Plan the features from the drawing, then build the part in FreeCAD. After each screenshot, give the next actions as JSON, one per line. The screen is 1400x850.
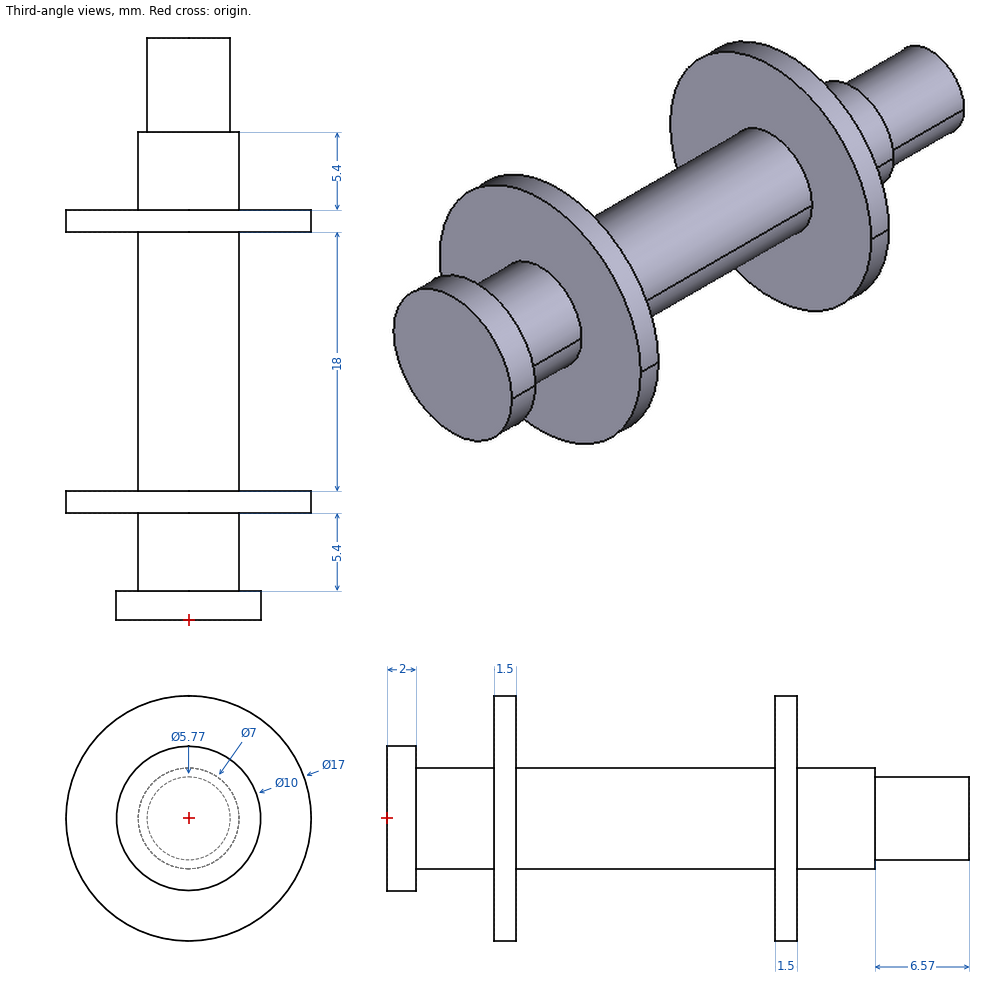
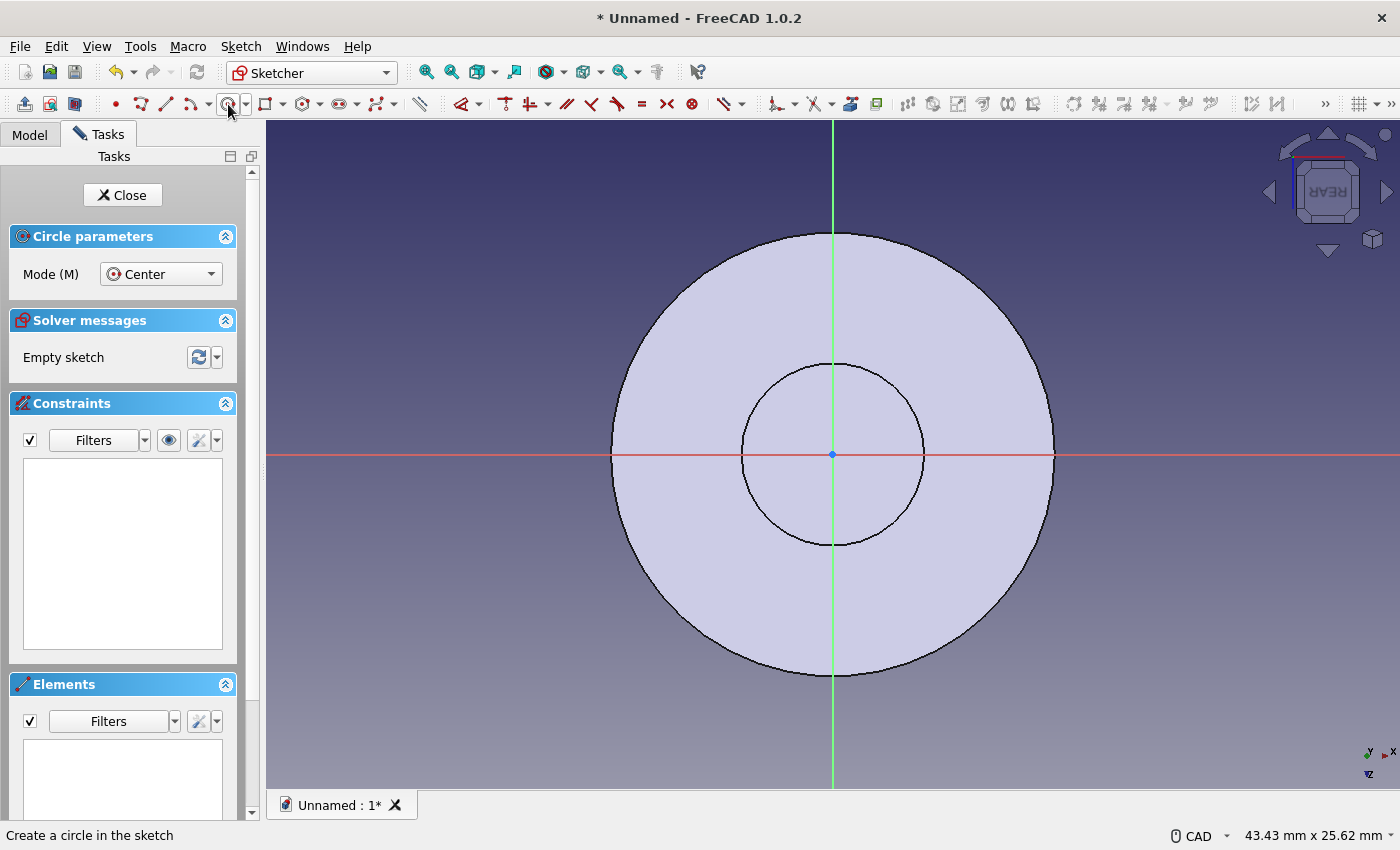
{"action": "left_click", "coordinate": [833, 455]}
{"action": "left_click", "coordinate": [990, 298]}
{"action": "key", "text": "Escape"}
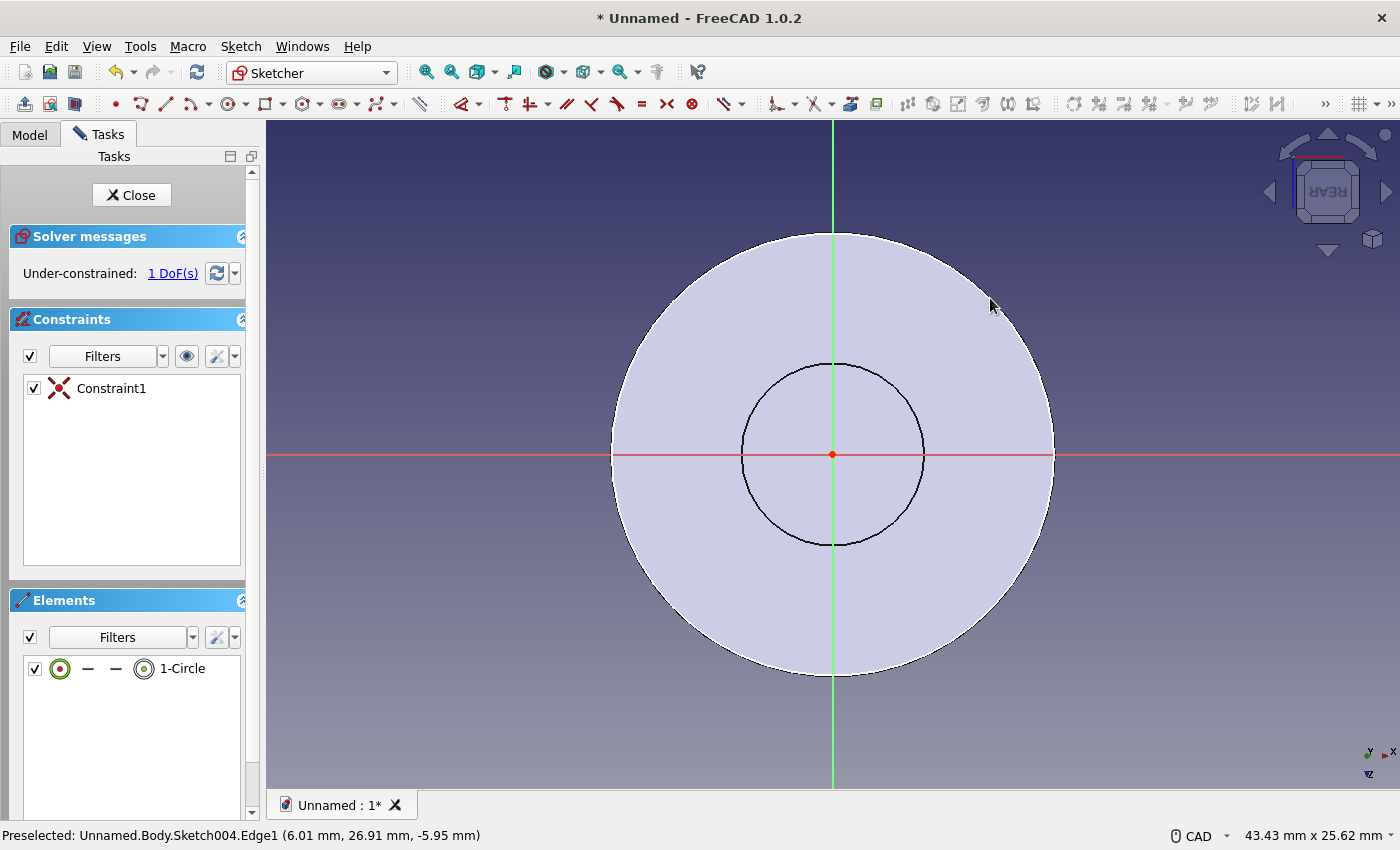
{"action": "left_click", "coordinate": [460, 104]}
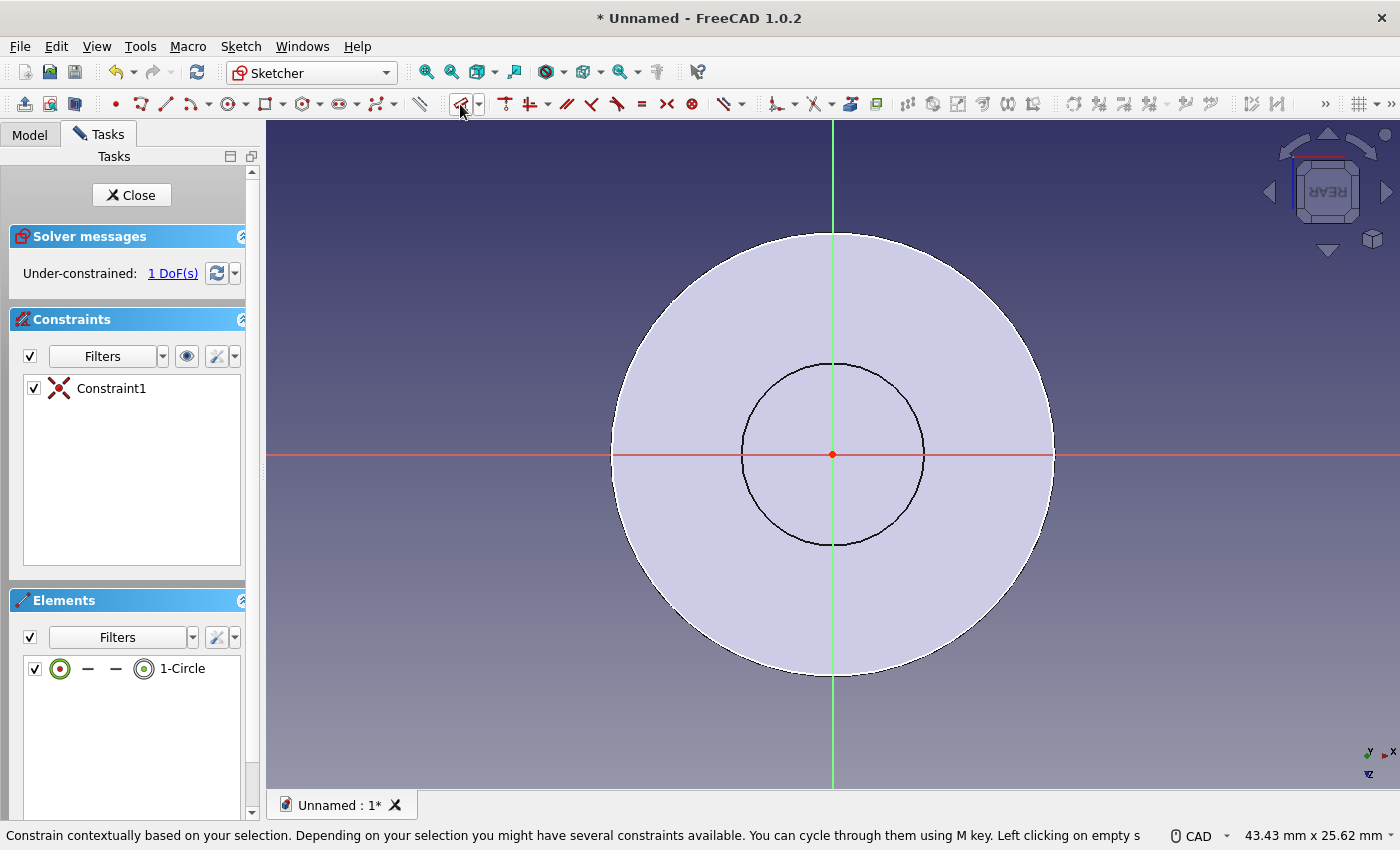
{"action": "left_click", "coordinate": [989, 298]}
{"action": "left_click", "coordinate": [1012, 275]}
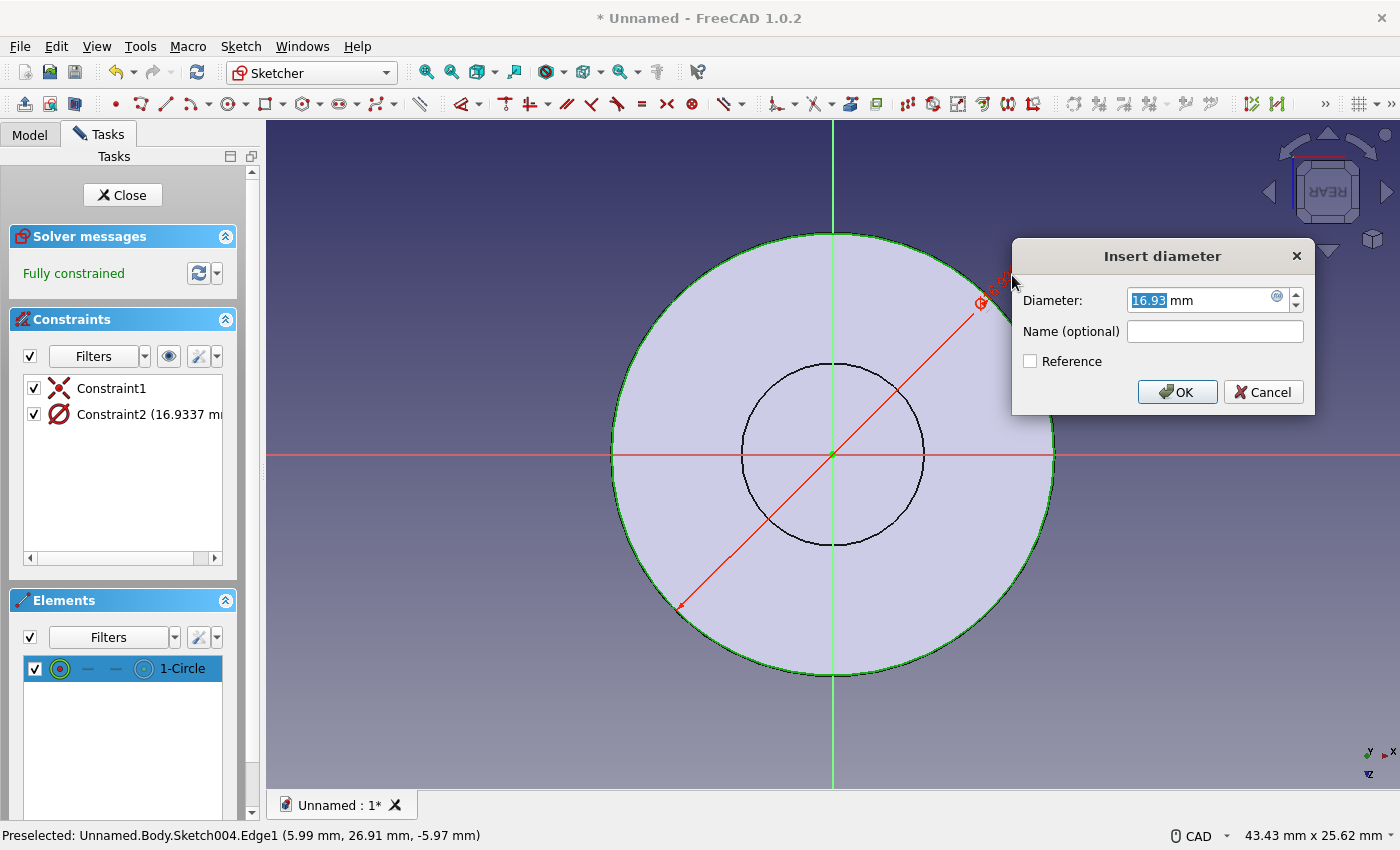
{"action": "type", "text": "17"}
{"action": "key", "text": "Return"}
{"action": "key", "text": "Escape"}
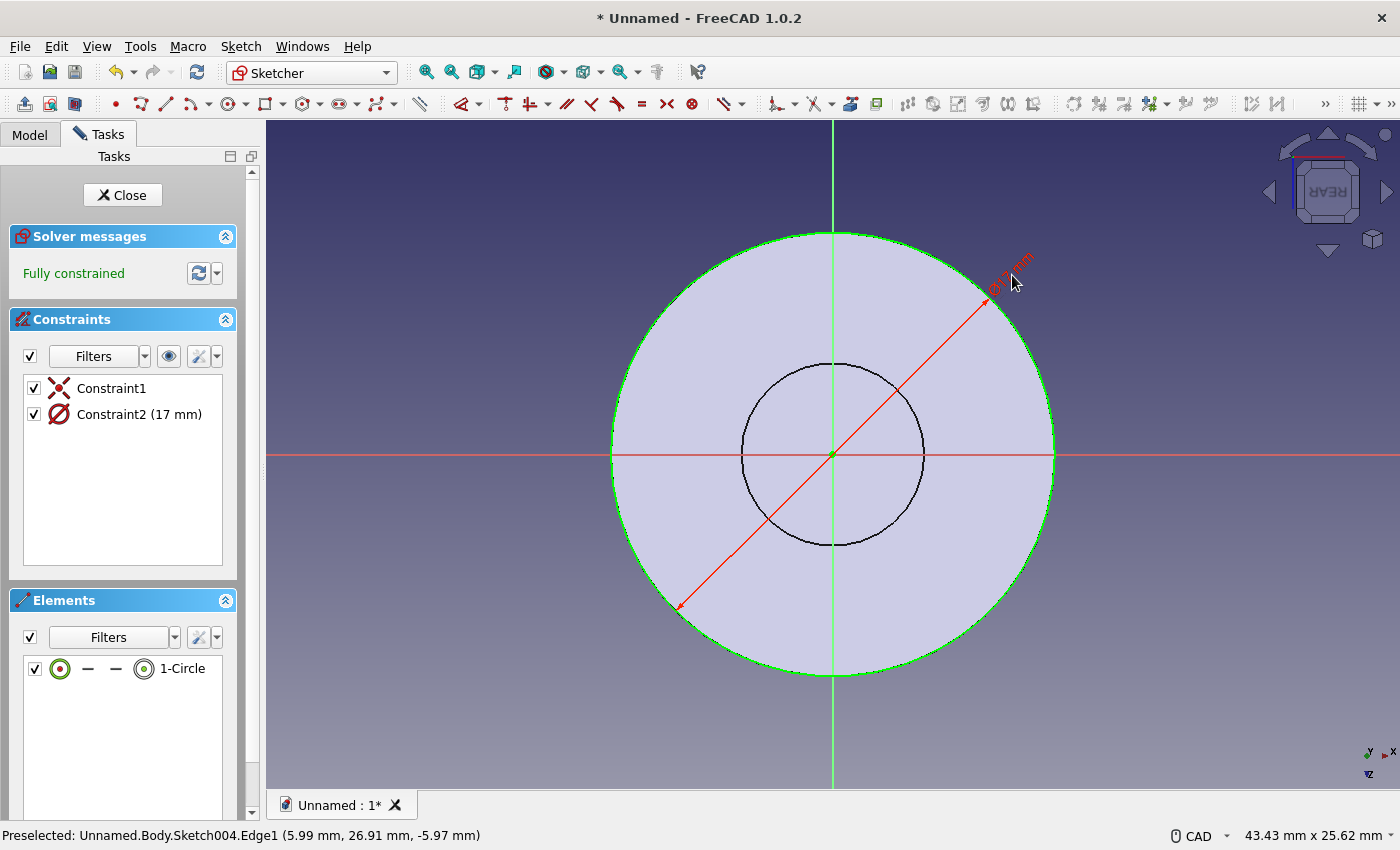
{"action": "left_click", "coordinate": [123, 195]}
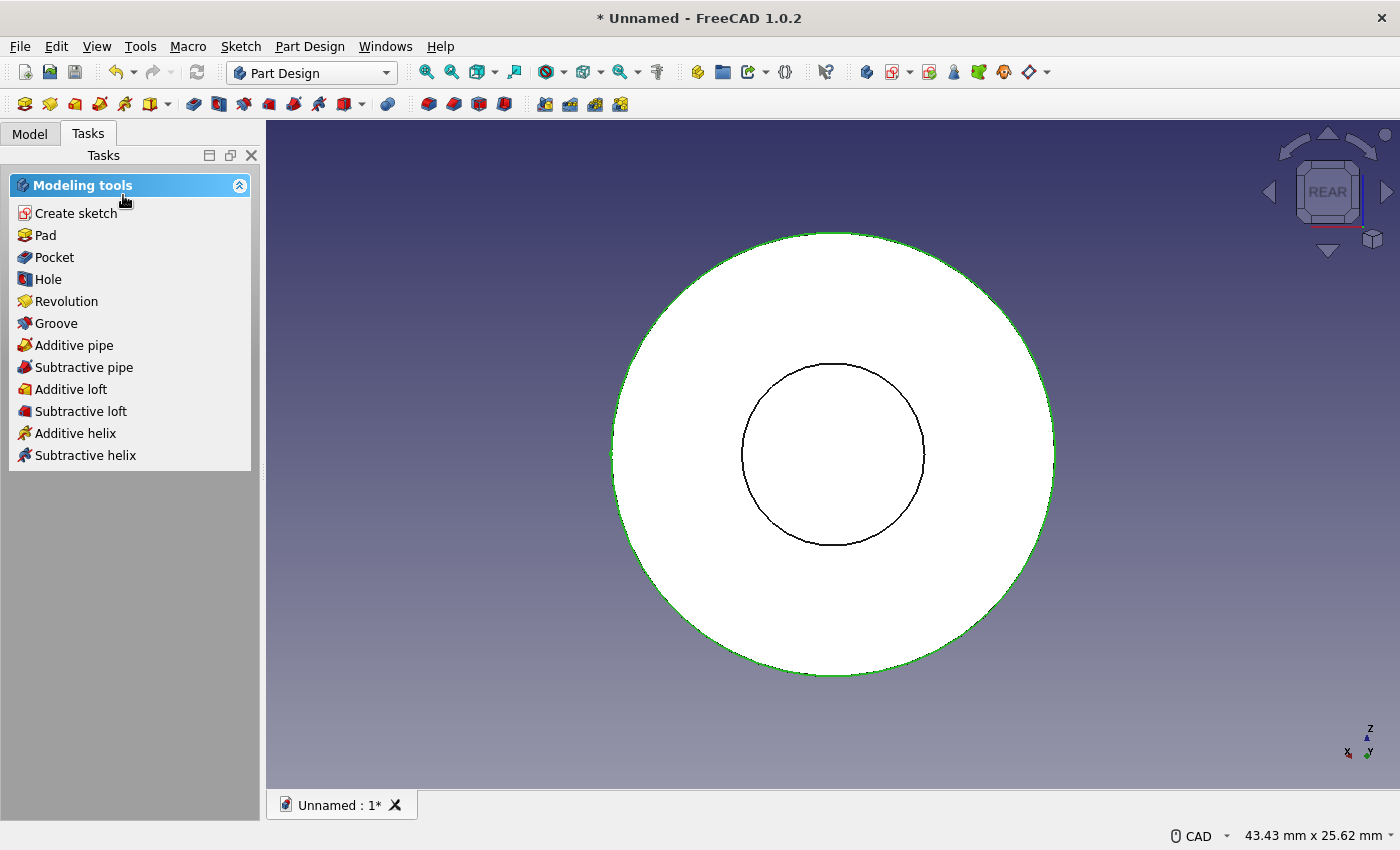
{"action": "left_click", "coordinate": [25, 104]}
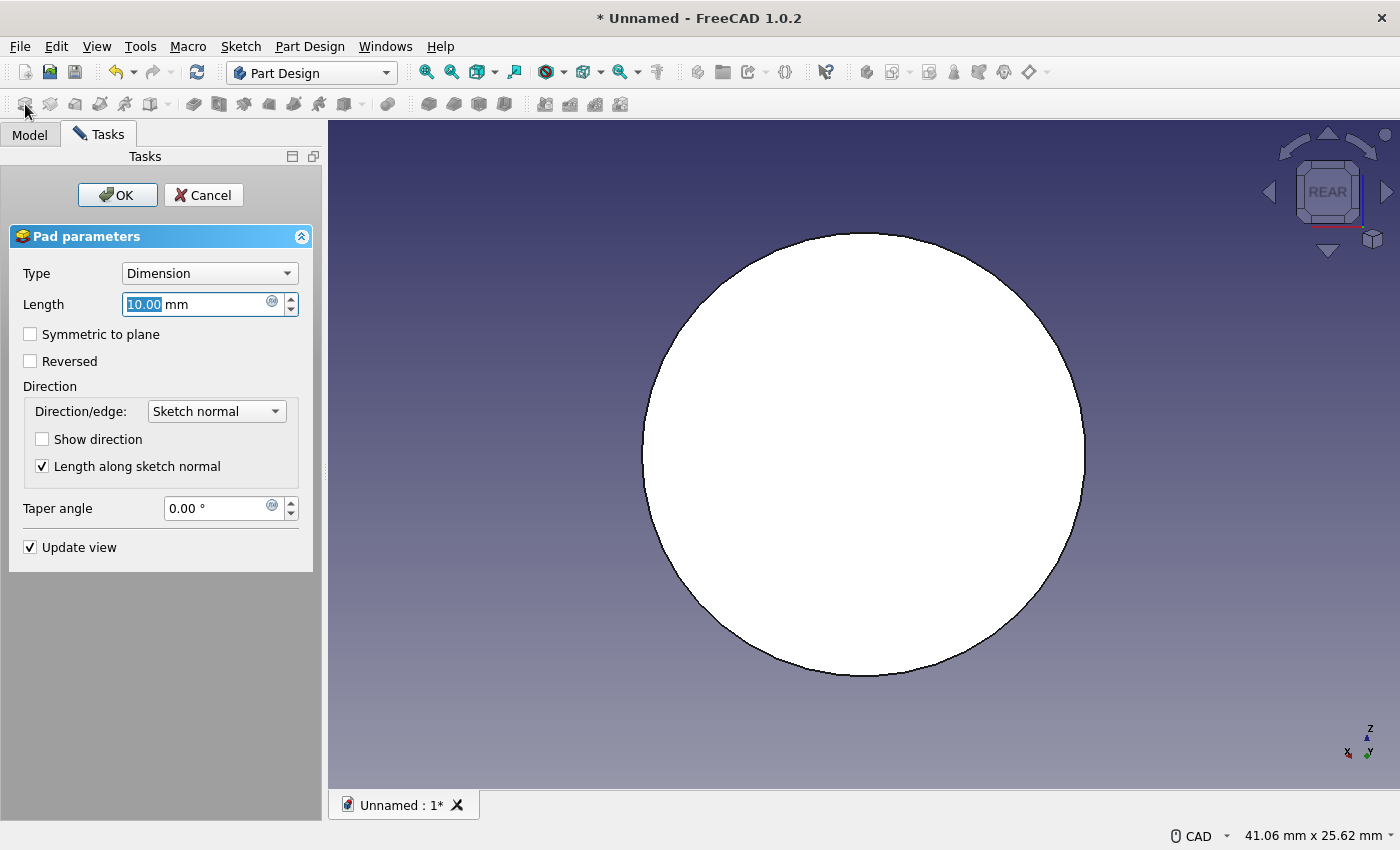
{"action": "type", "text": "1.5"}
{"action": "key", "text": "Tab"}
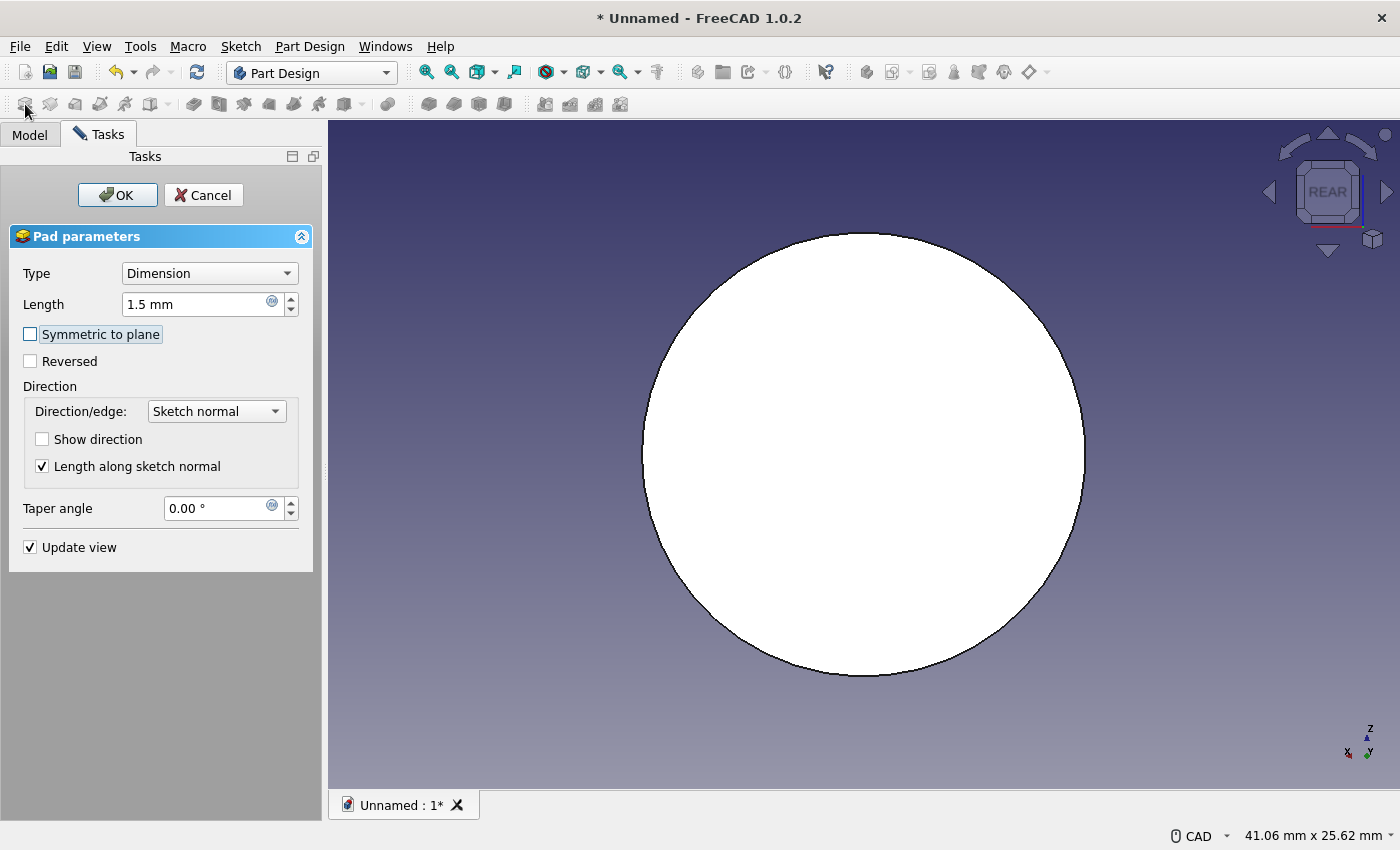
{"action": "left_click", "coordinate": [118, 195]}